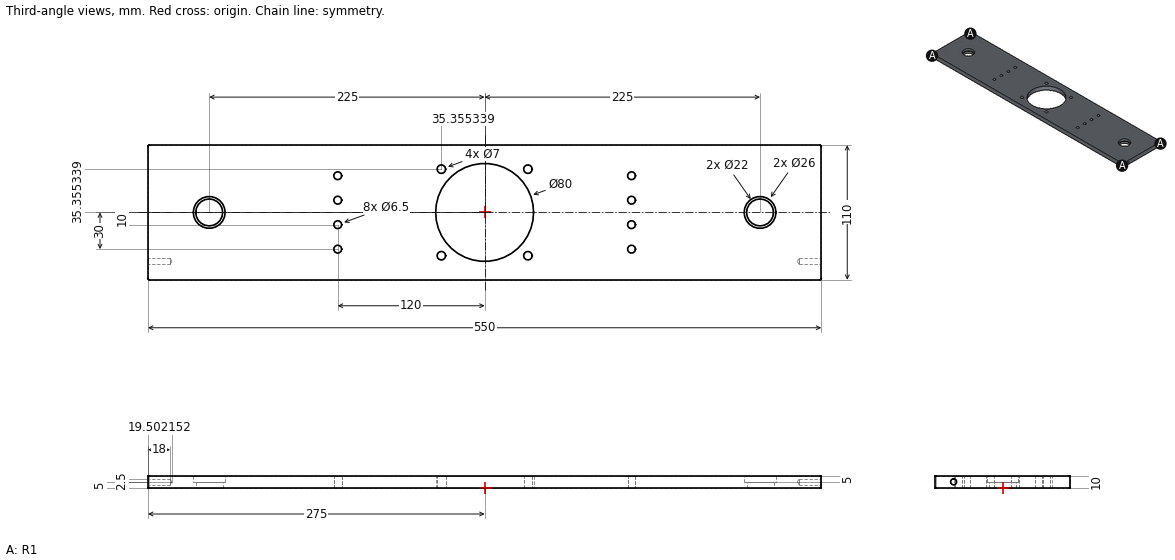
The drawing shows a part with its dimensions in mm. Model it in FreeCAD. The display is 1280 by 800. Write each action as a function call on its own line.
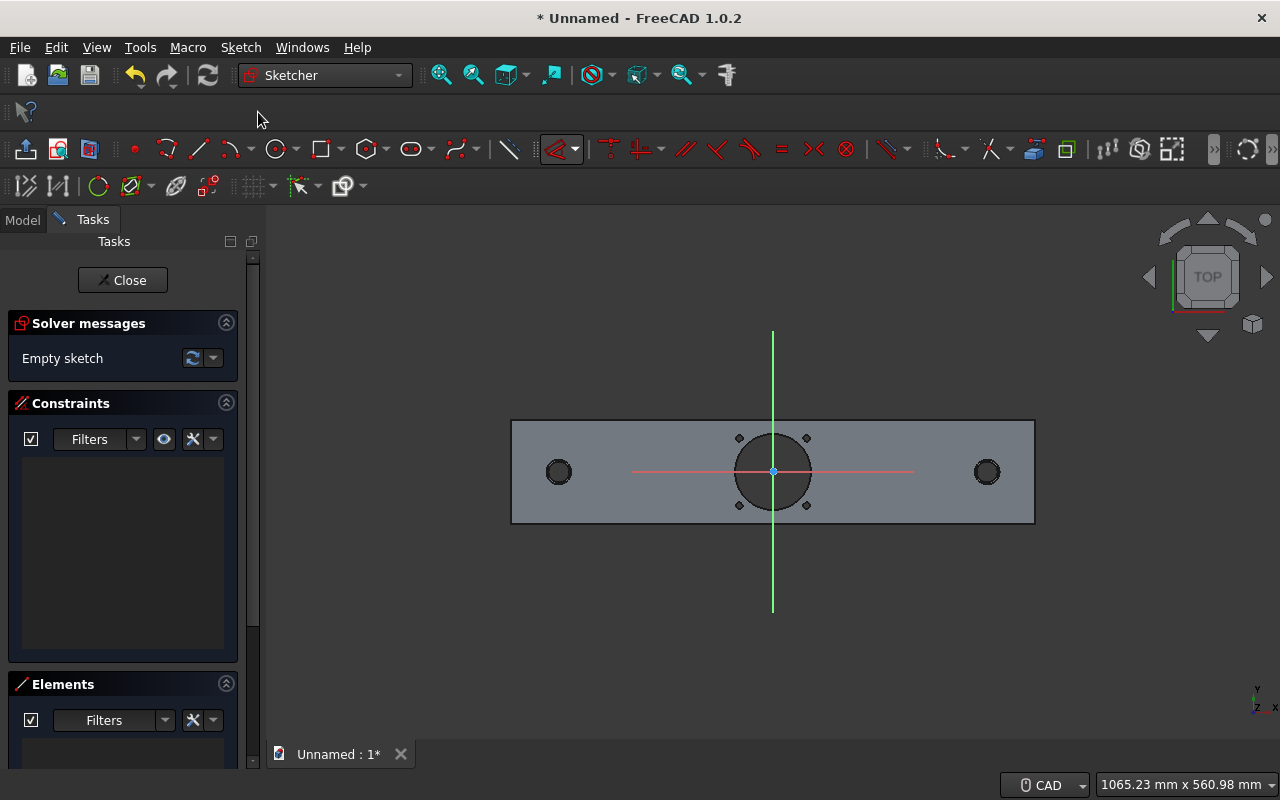
scroll(813, 472, up, 5)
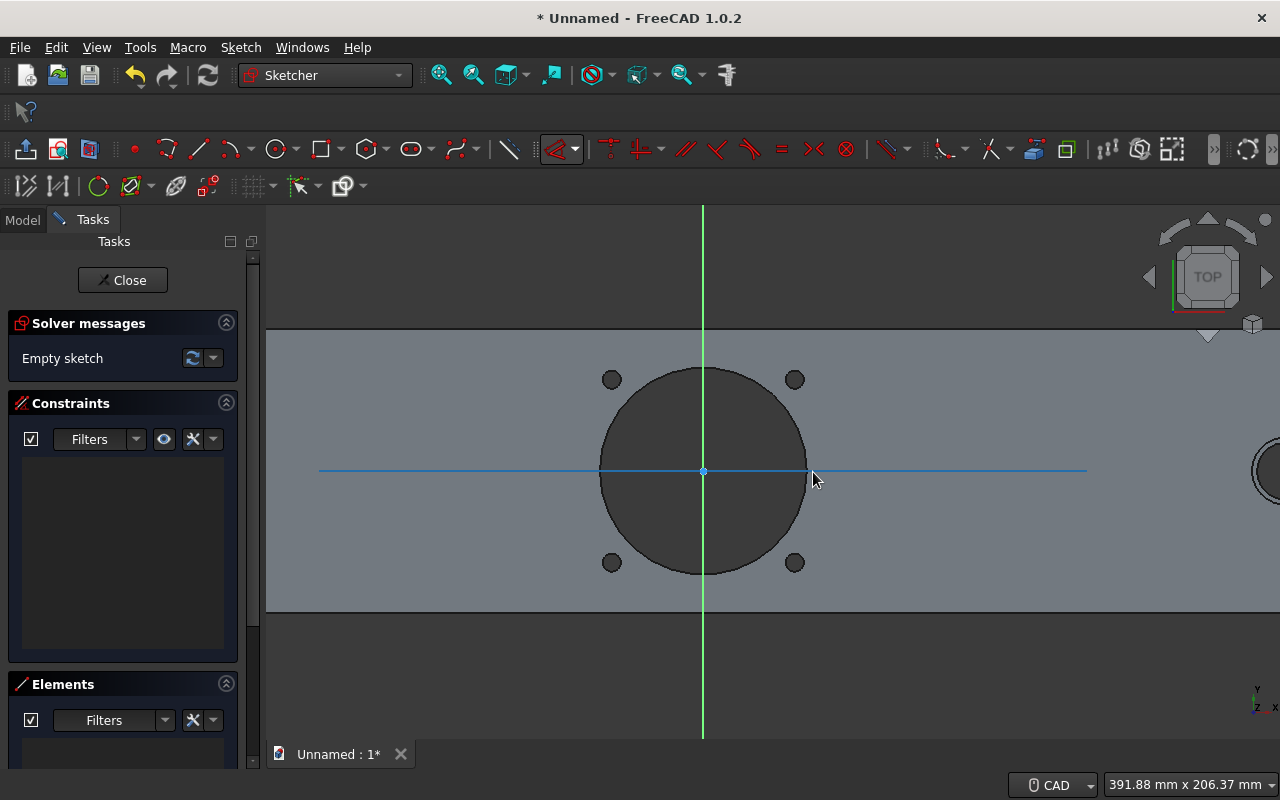
click(276, 150)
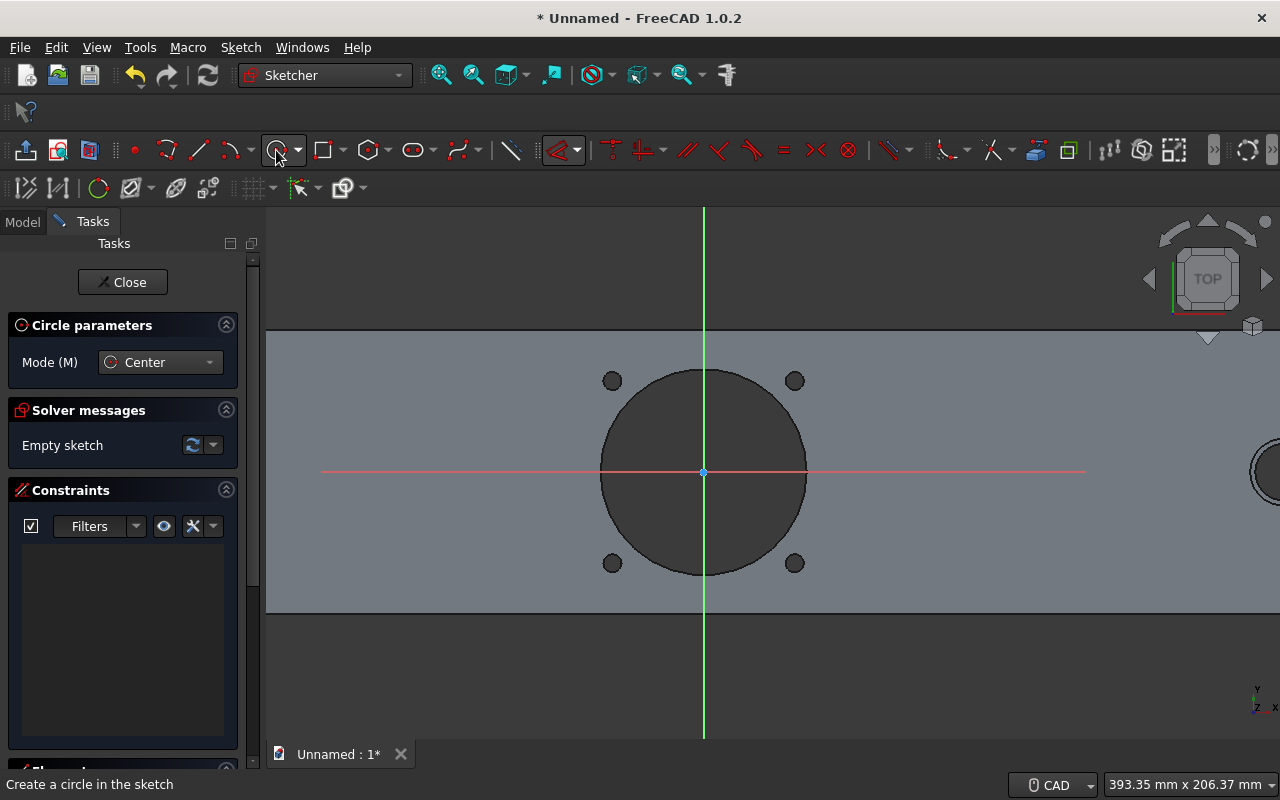
scroll(394, 498, up, 5)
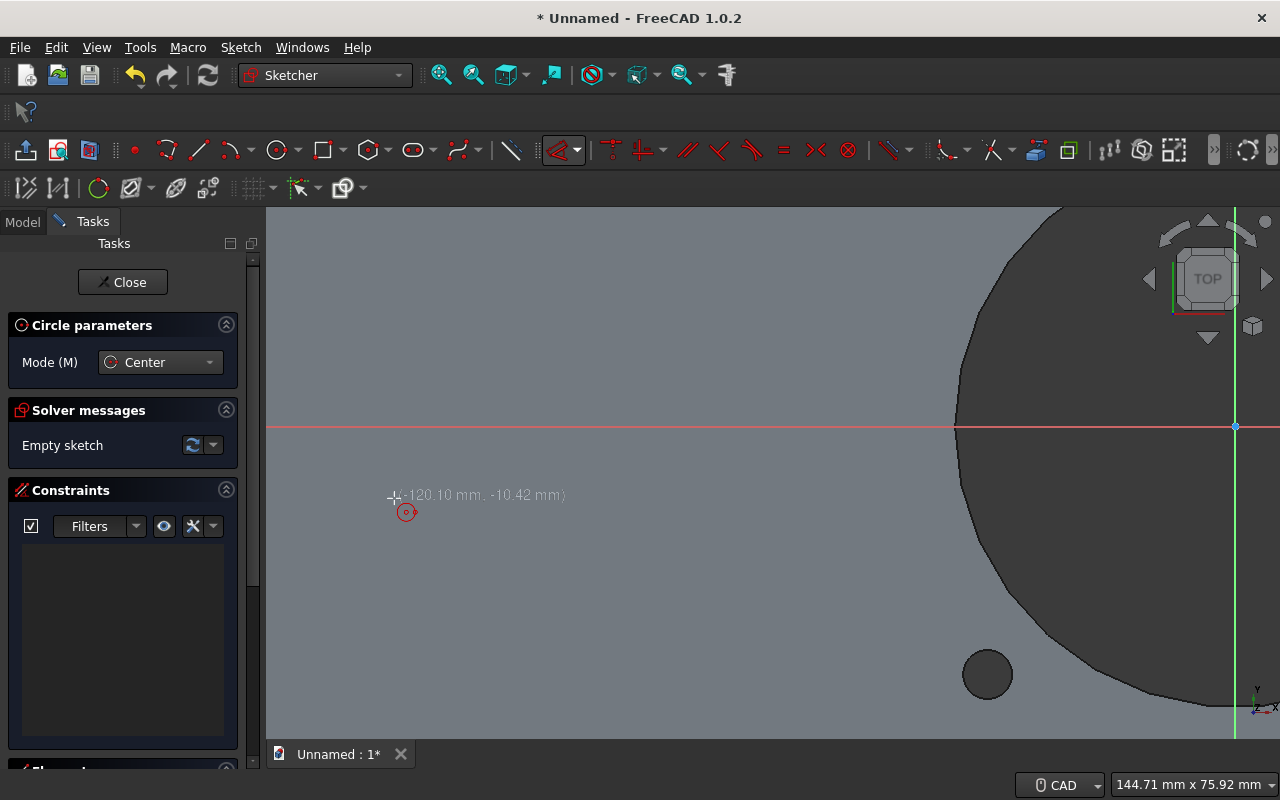
click(394, 497)
move(411, 481)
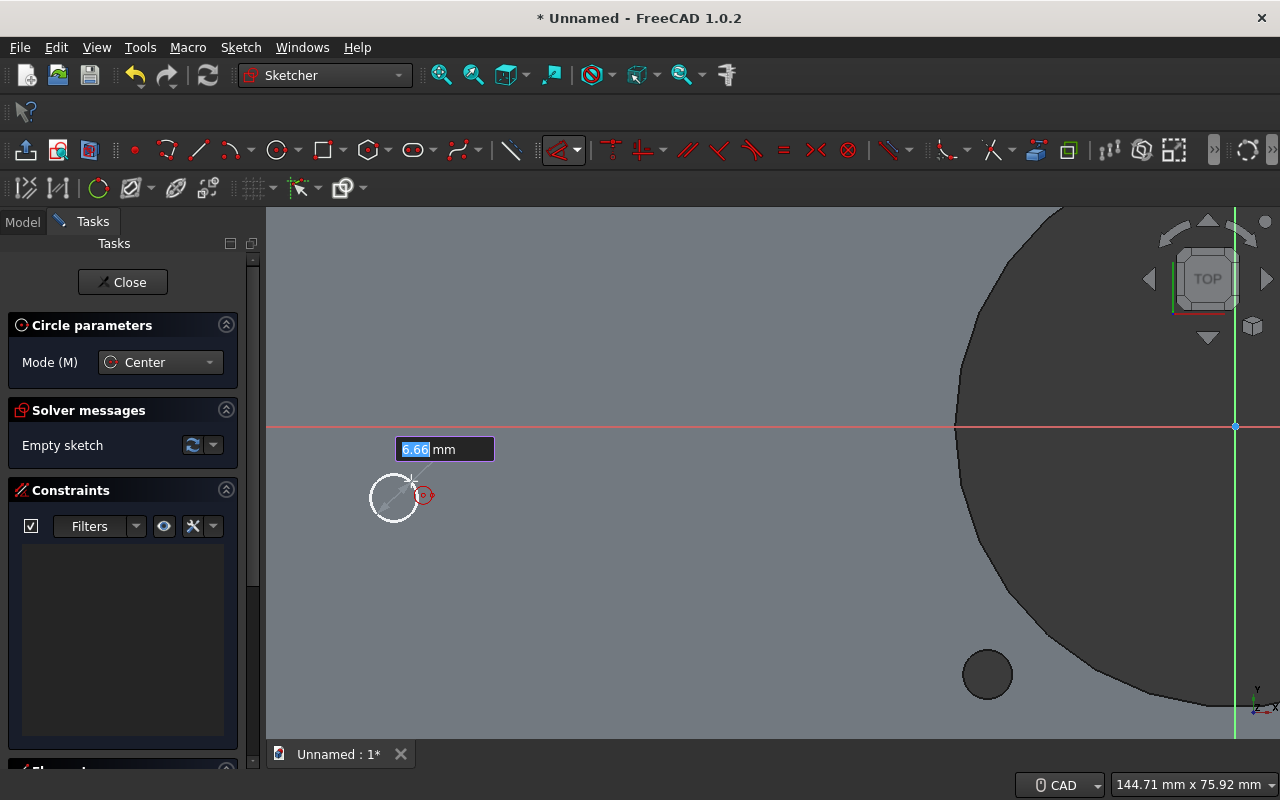
text(6.5)
key(Return)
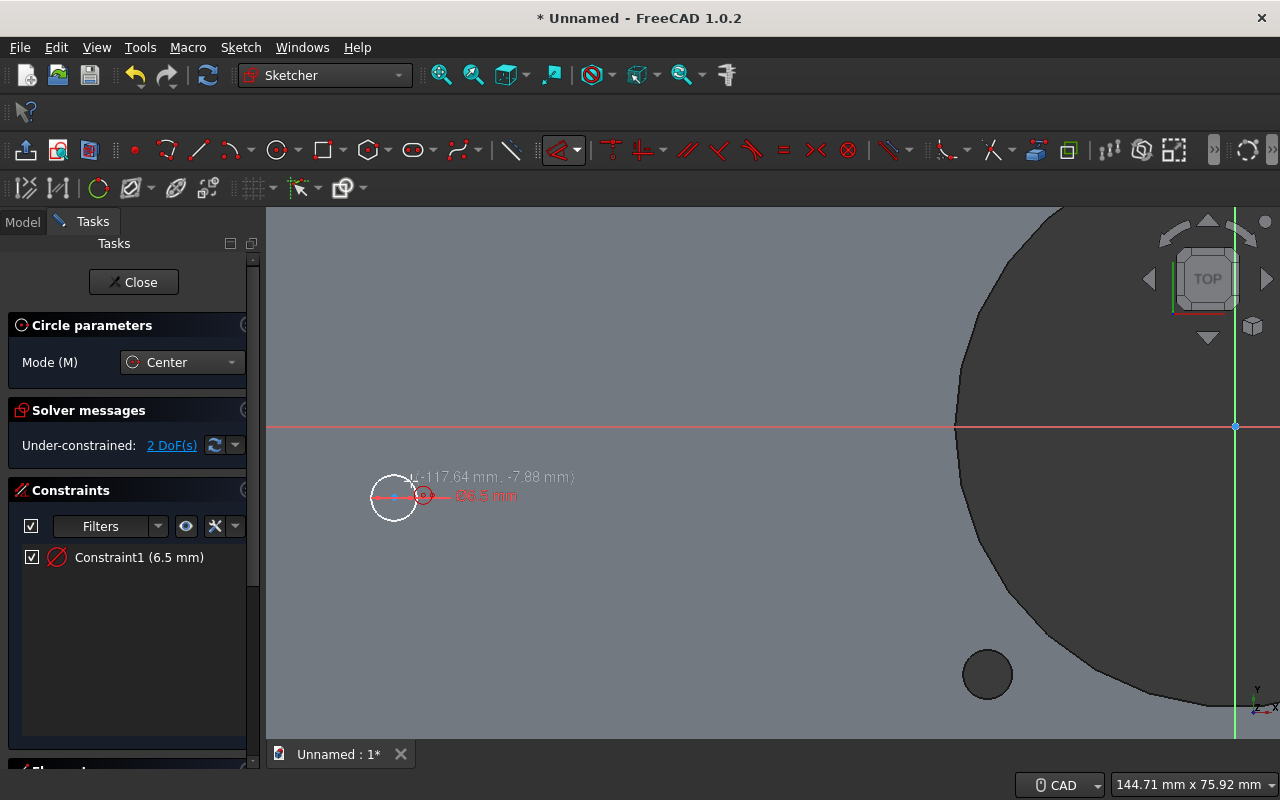
scroll(396, 500, down, 5)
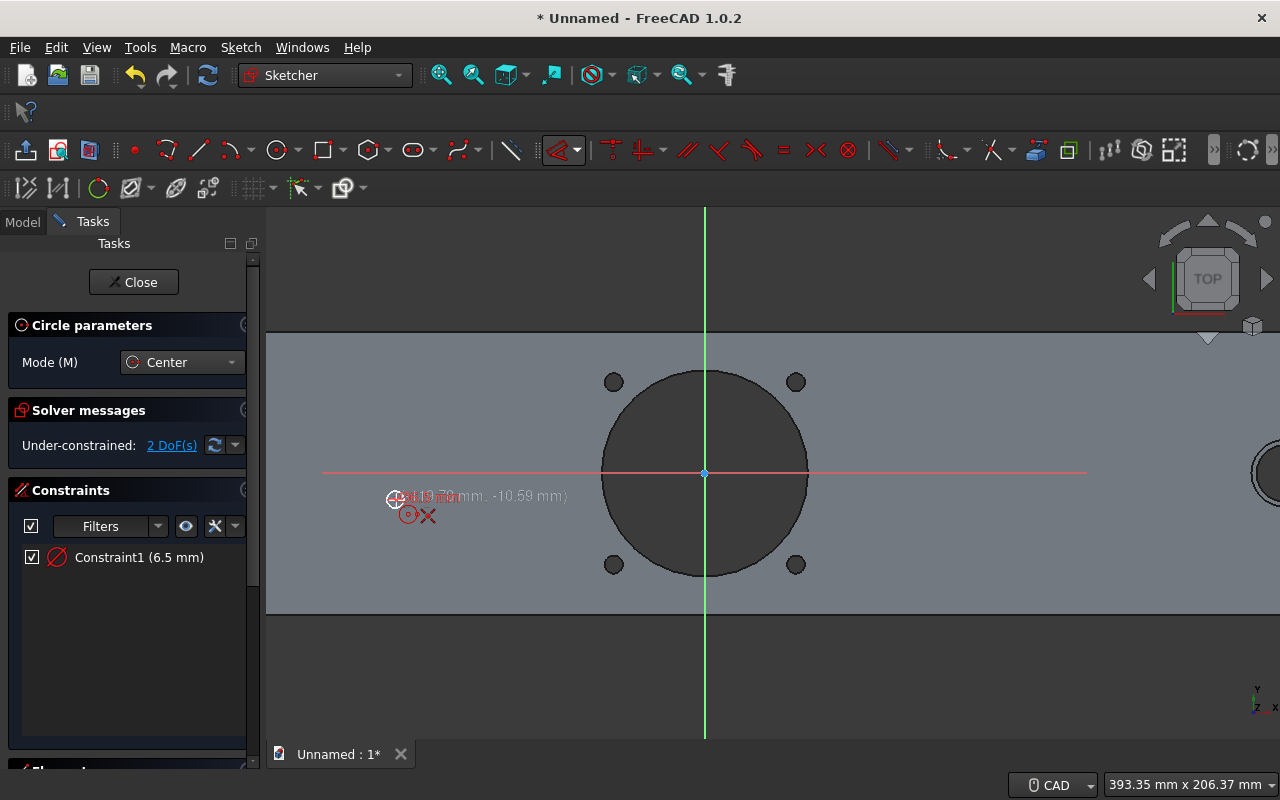
scroll(1014, 499, up, 5)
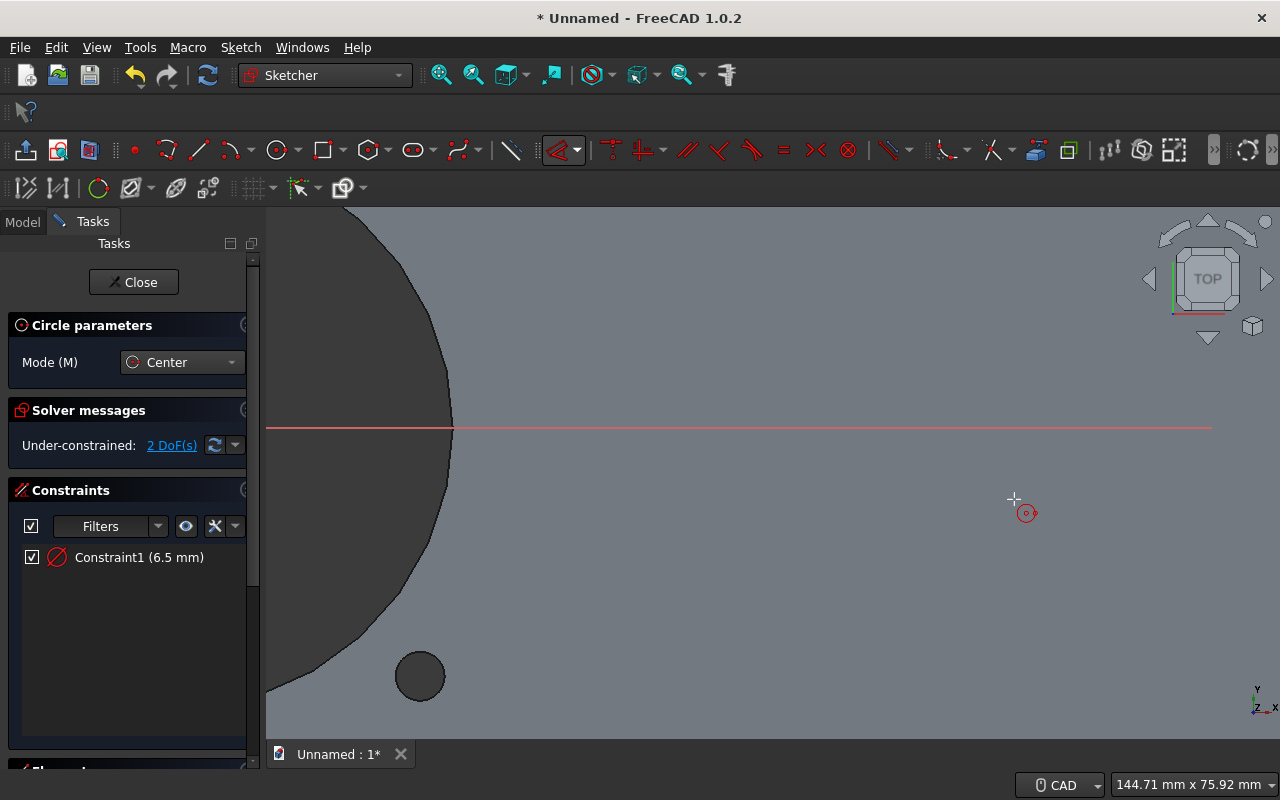
click(1013, 499)
move(1029, 482)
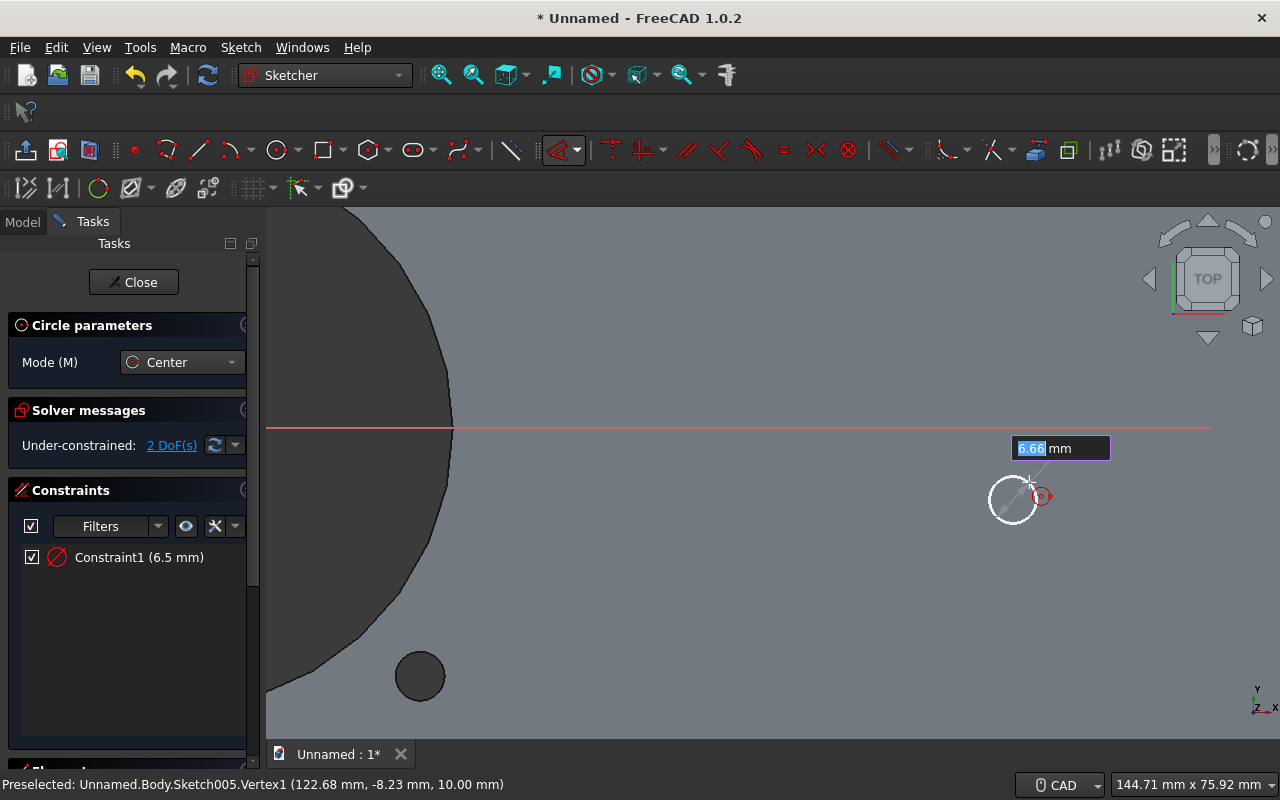
text(6.5)
key(Return)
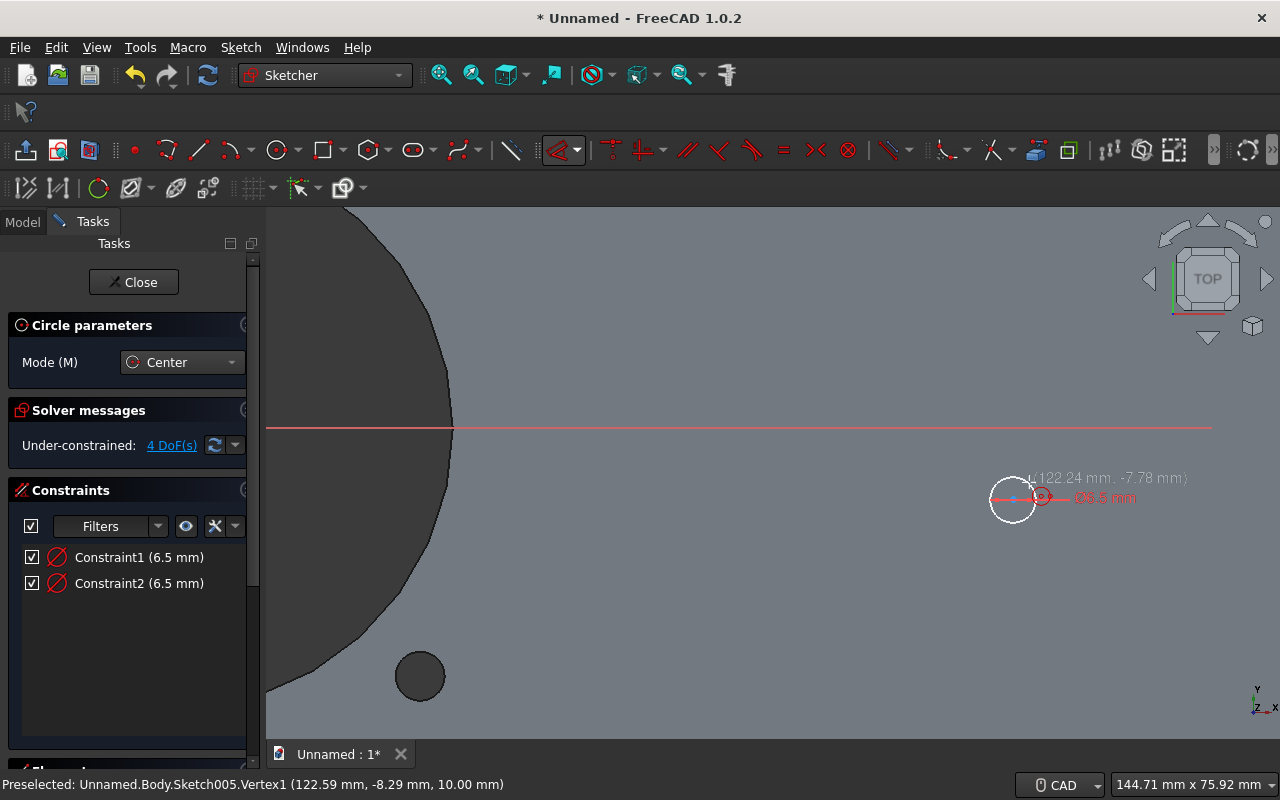
click(1013, 358)
move(1029, 342)